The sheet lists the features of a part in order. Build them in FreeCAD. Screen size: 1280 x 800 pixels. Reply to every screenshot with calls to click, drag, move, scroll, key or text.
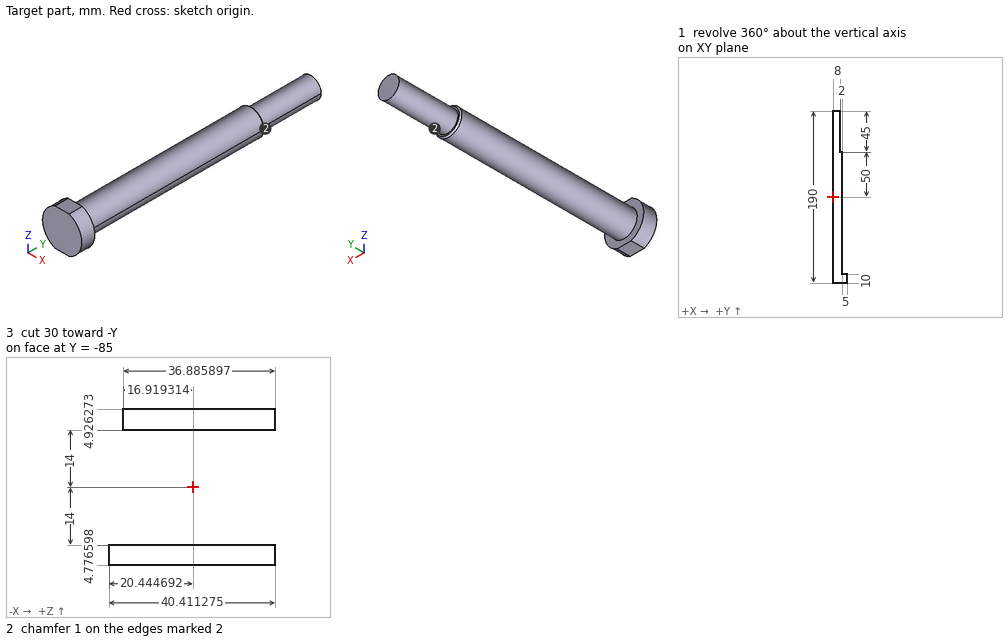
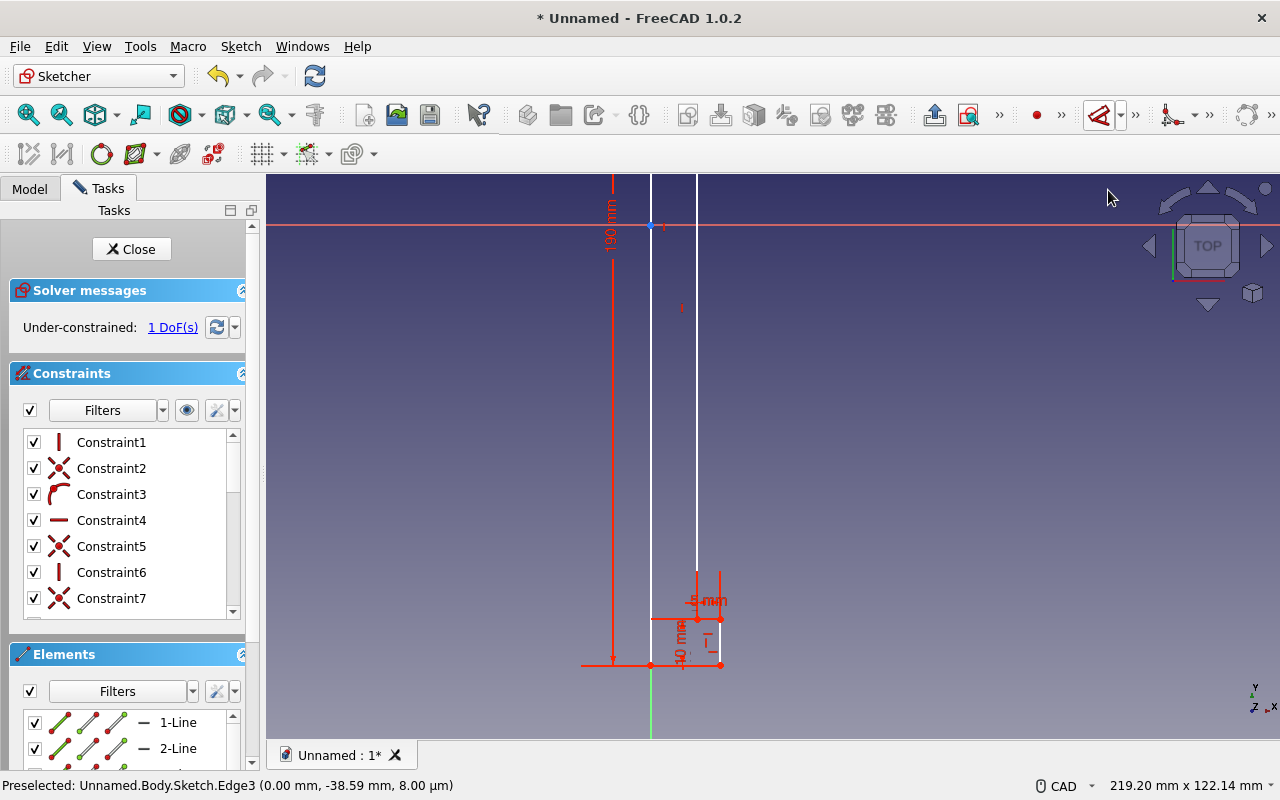
scroll(720, 645, down, 4)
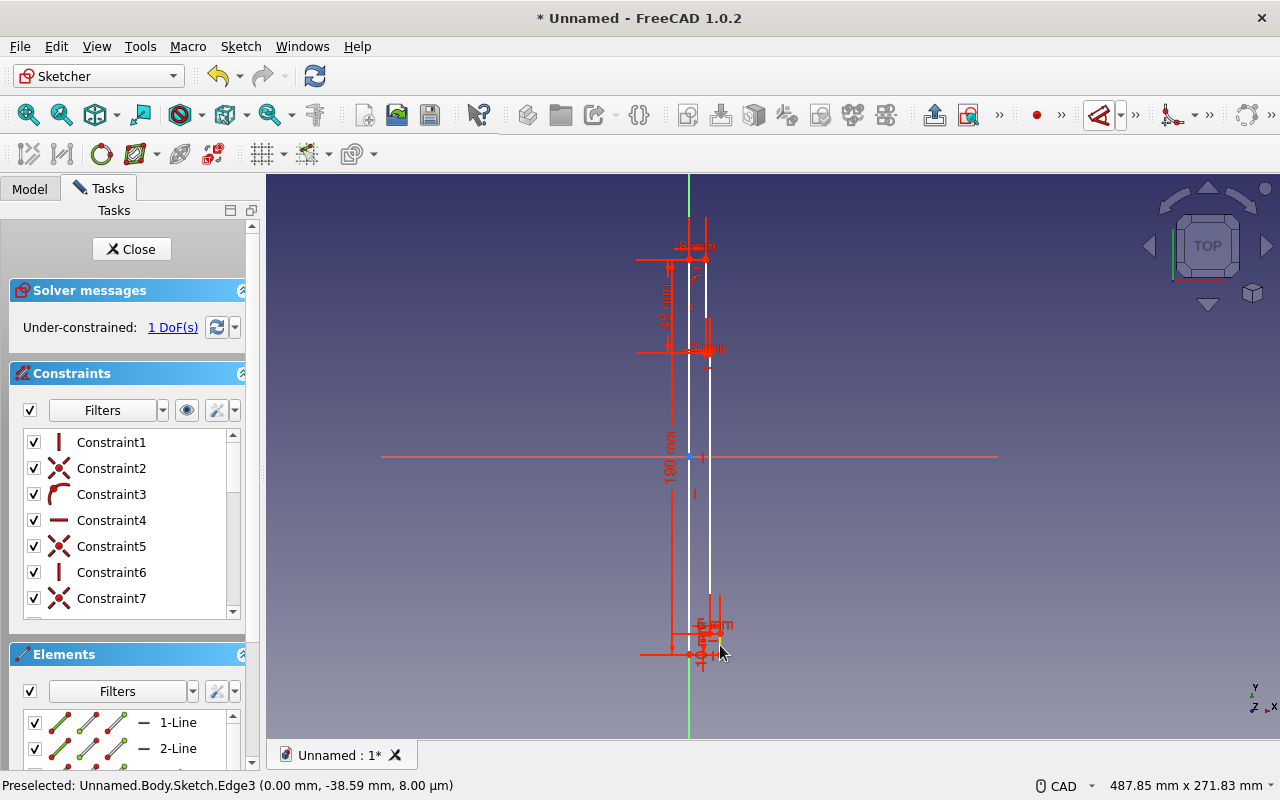
scroll(706, 353, up, 6)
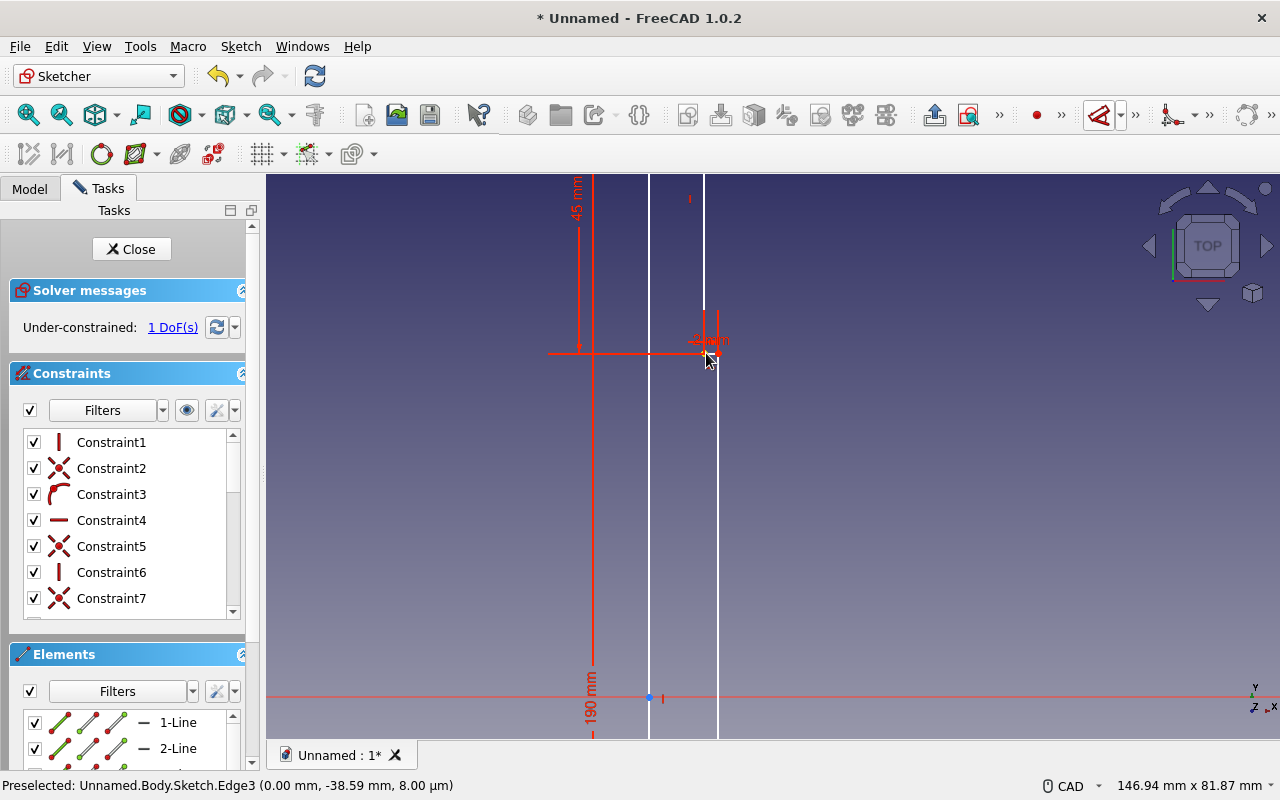
click(704, 354)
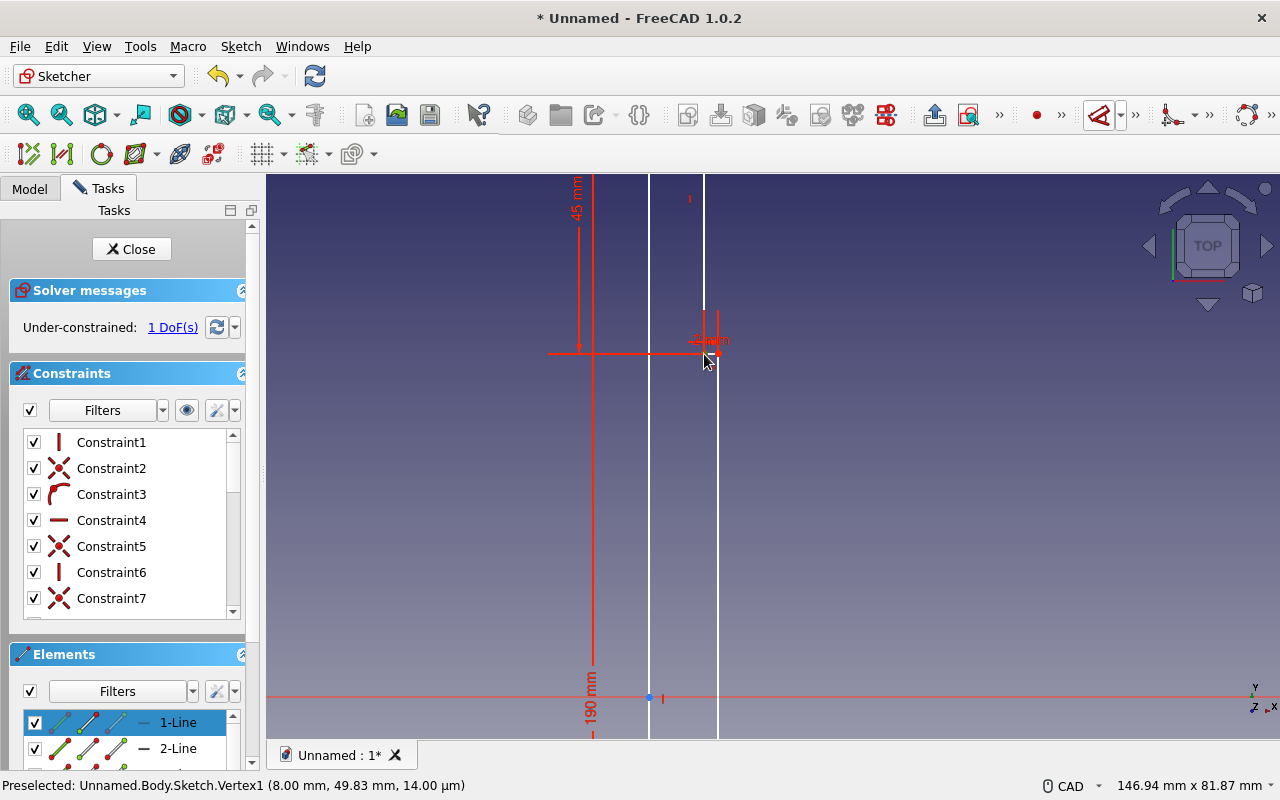
click(1120, 116)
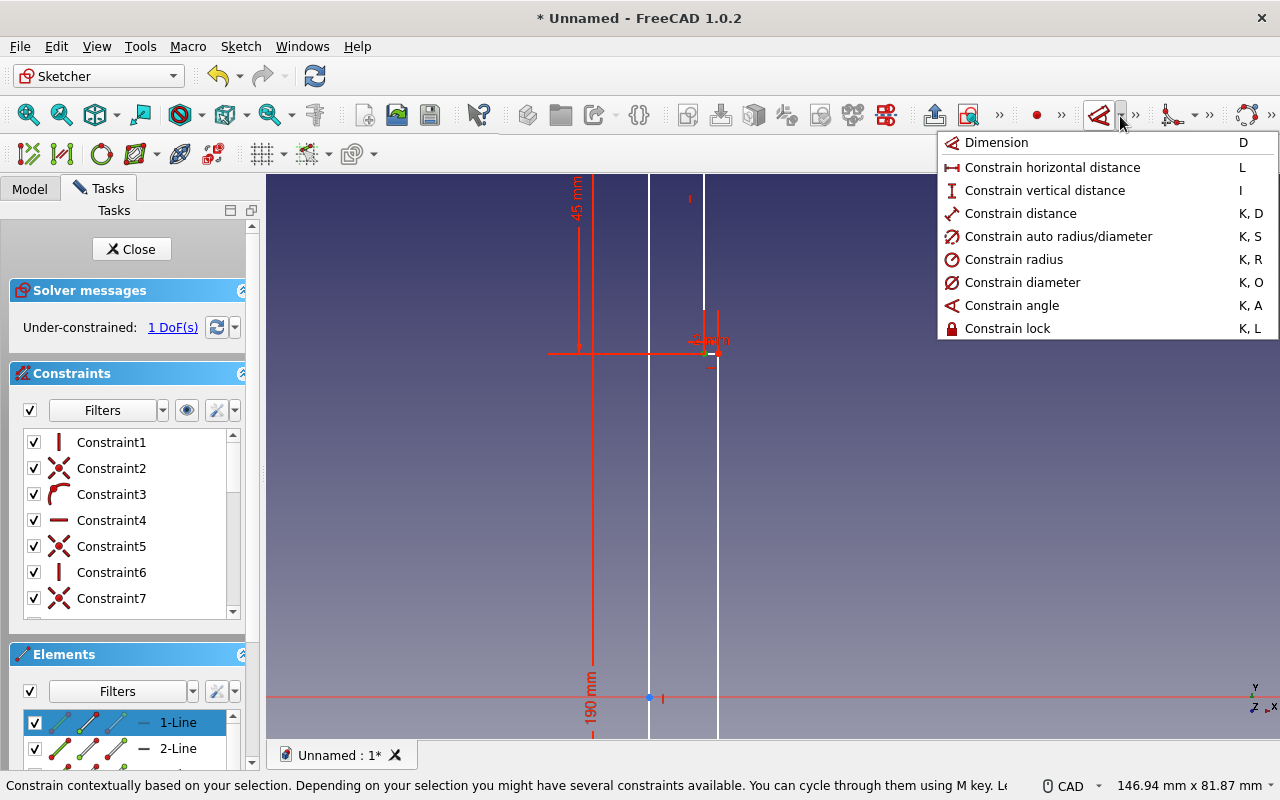
click(1108, 190)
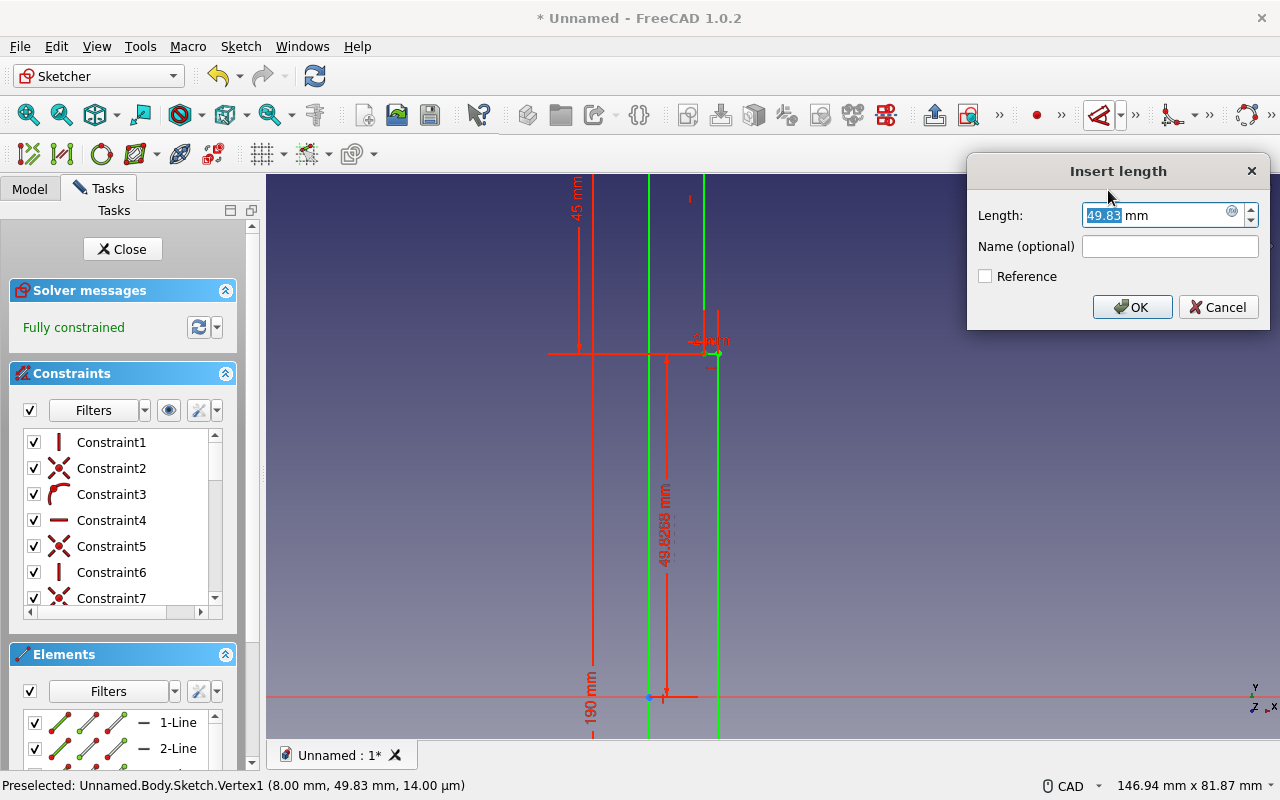
text(50)
key(Return)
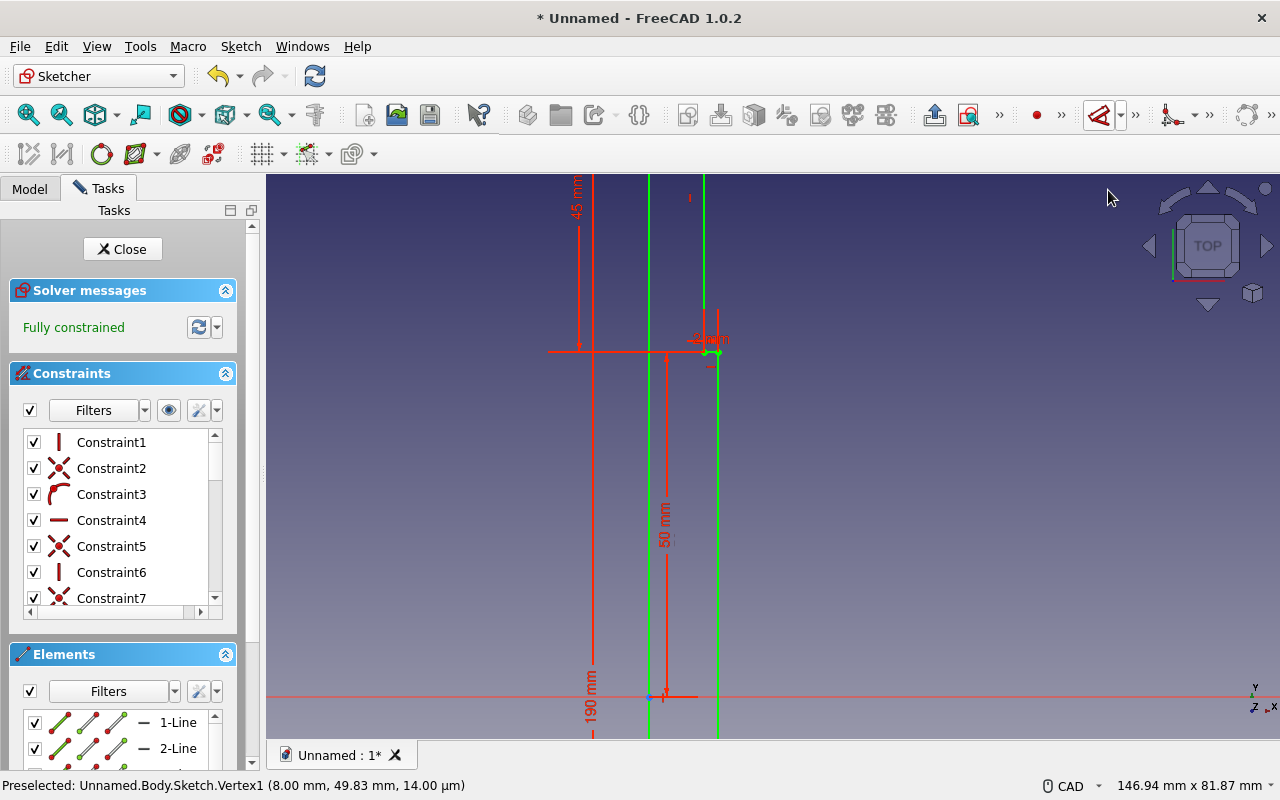
click(123, 249)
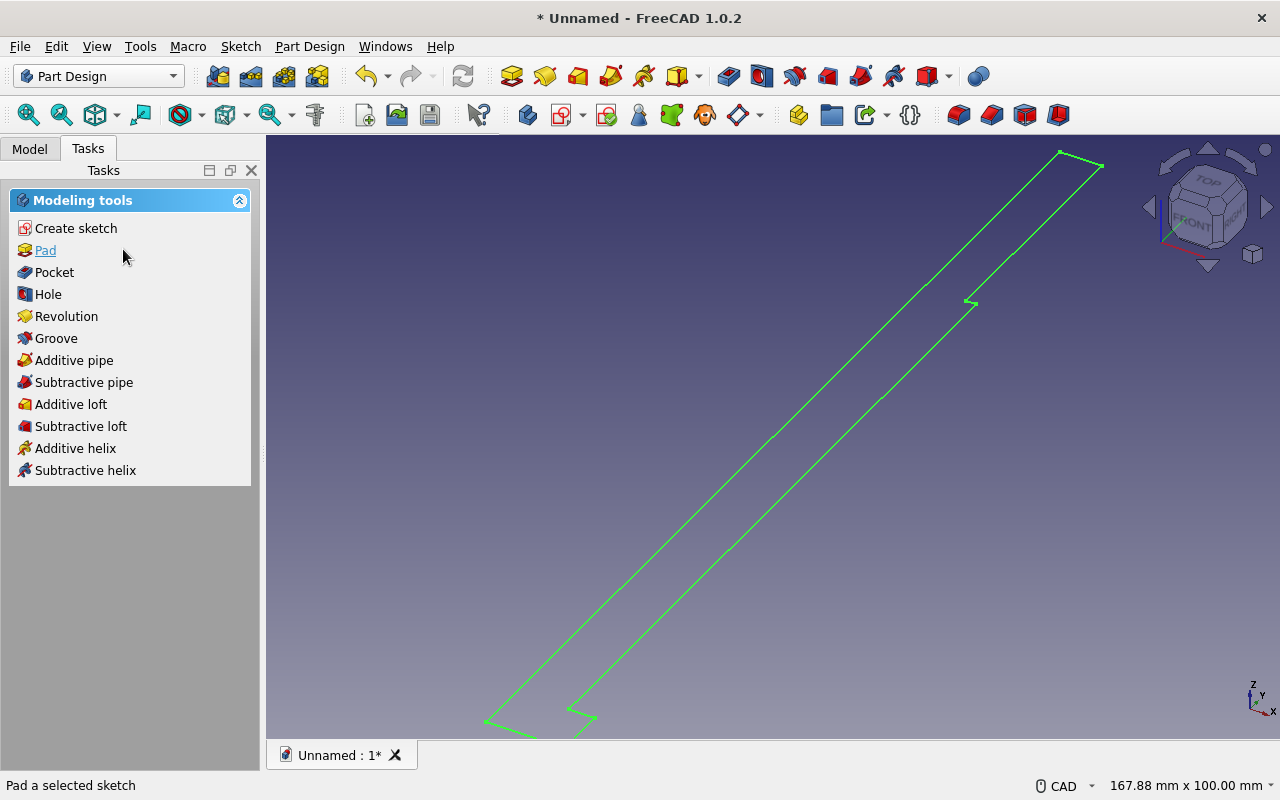
click(545, 76)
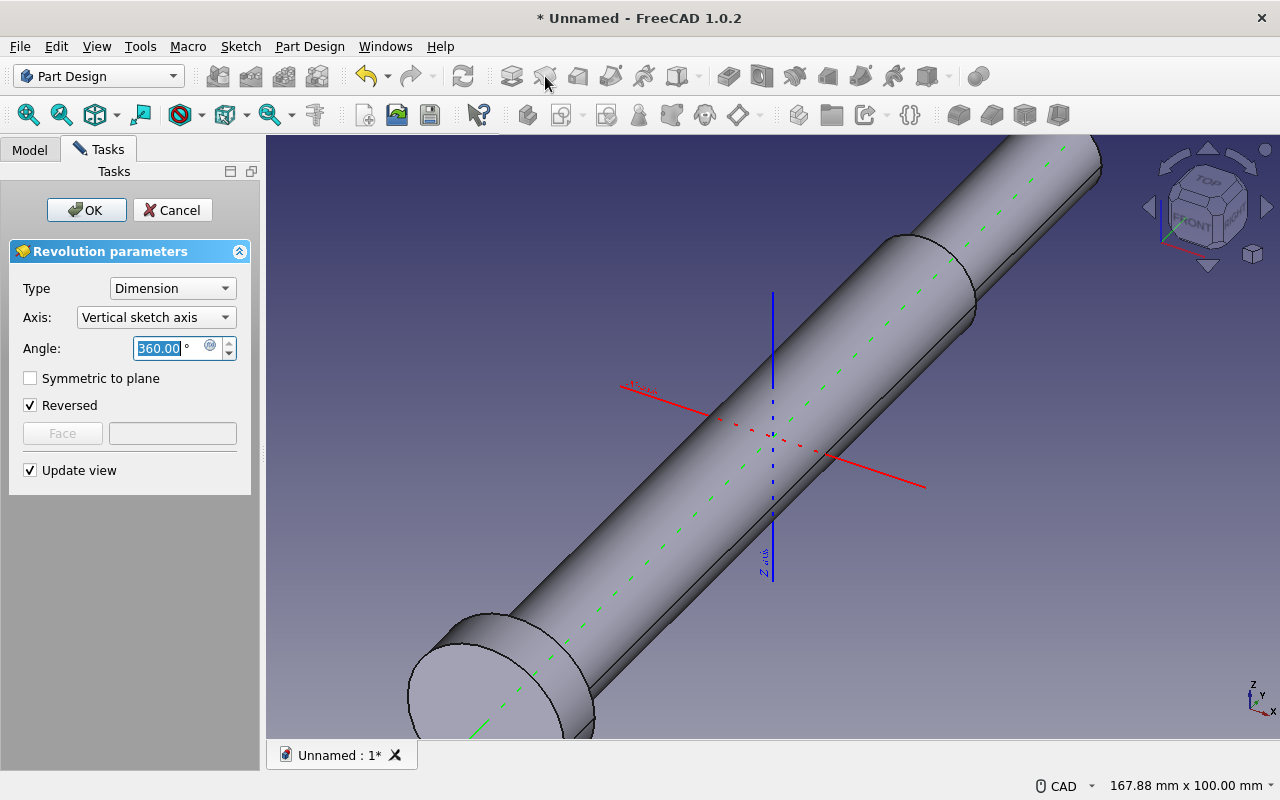
click(87, 210)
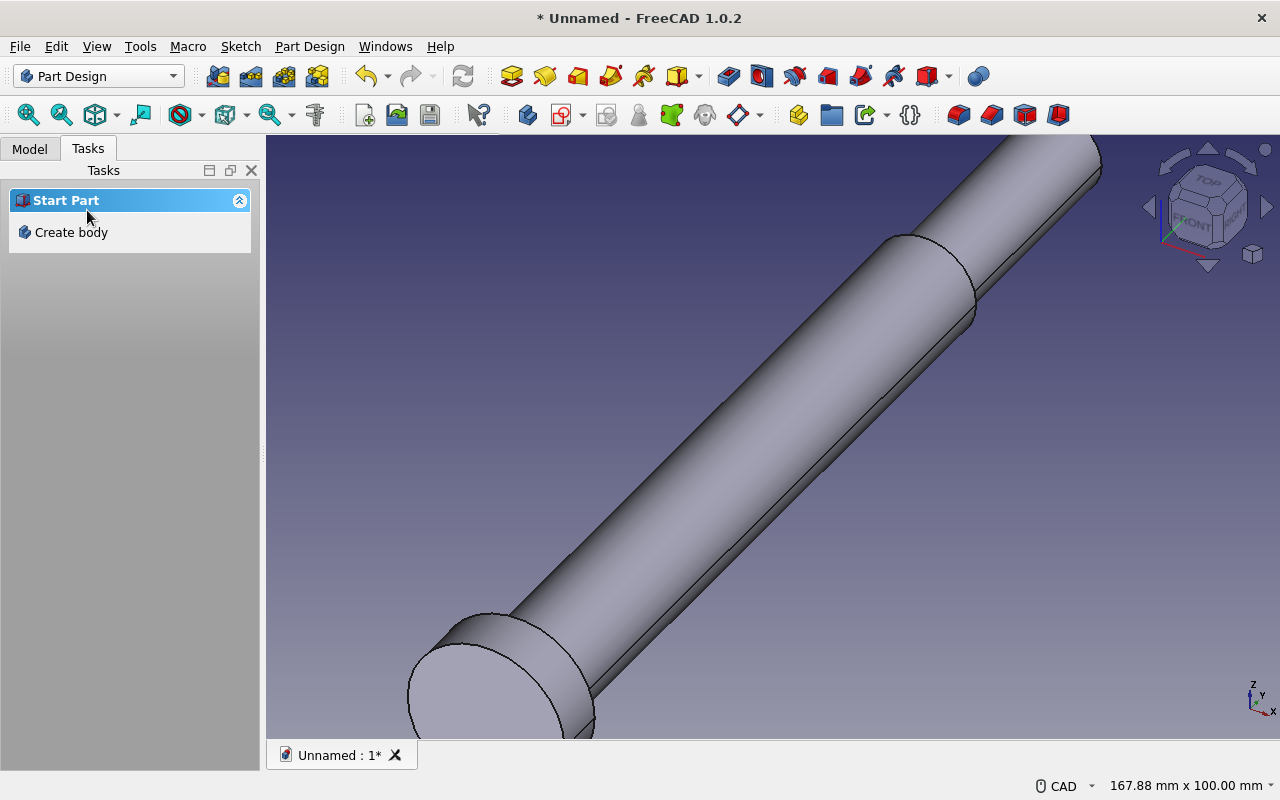
key(v)
key(f)